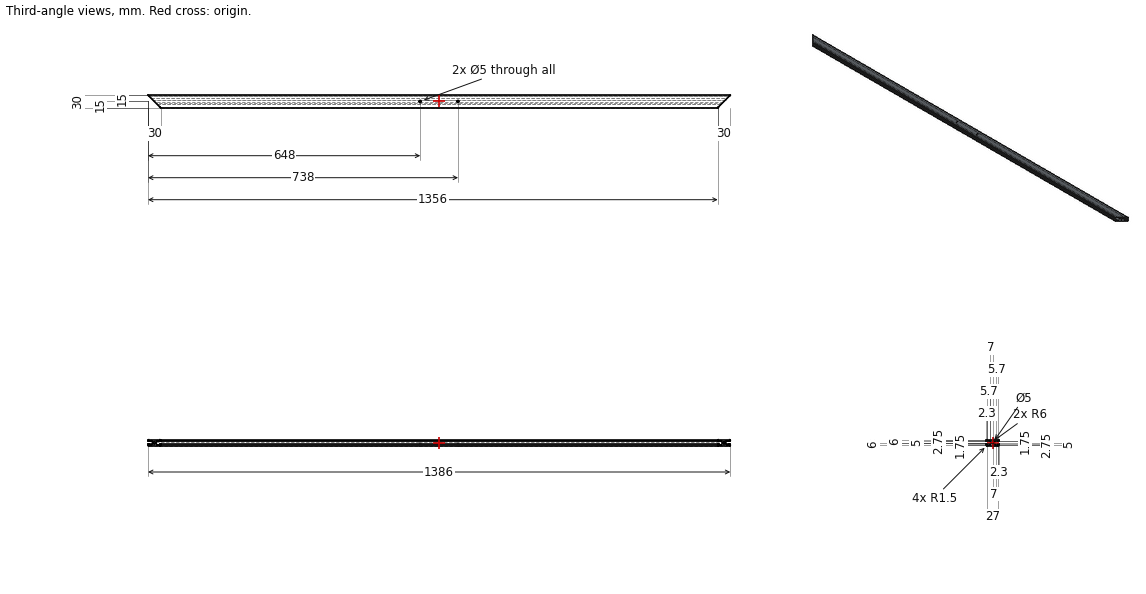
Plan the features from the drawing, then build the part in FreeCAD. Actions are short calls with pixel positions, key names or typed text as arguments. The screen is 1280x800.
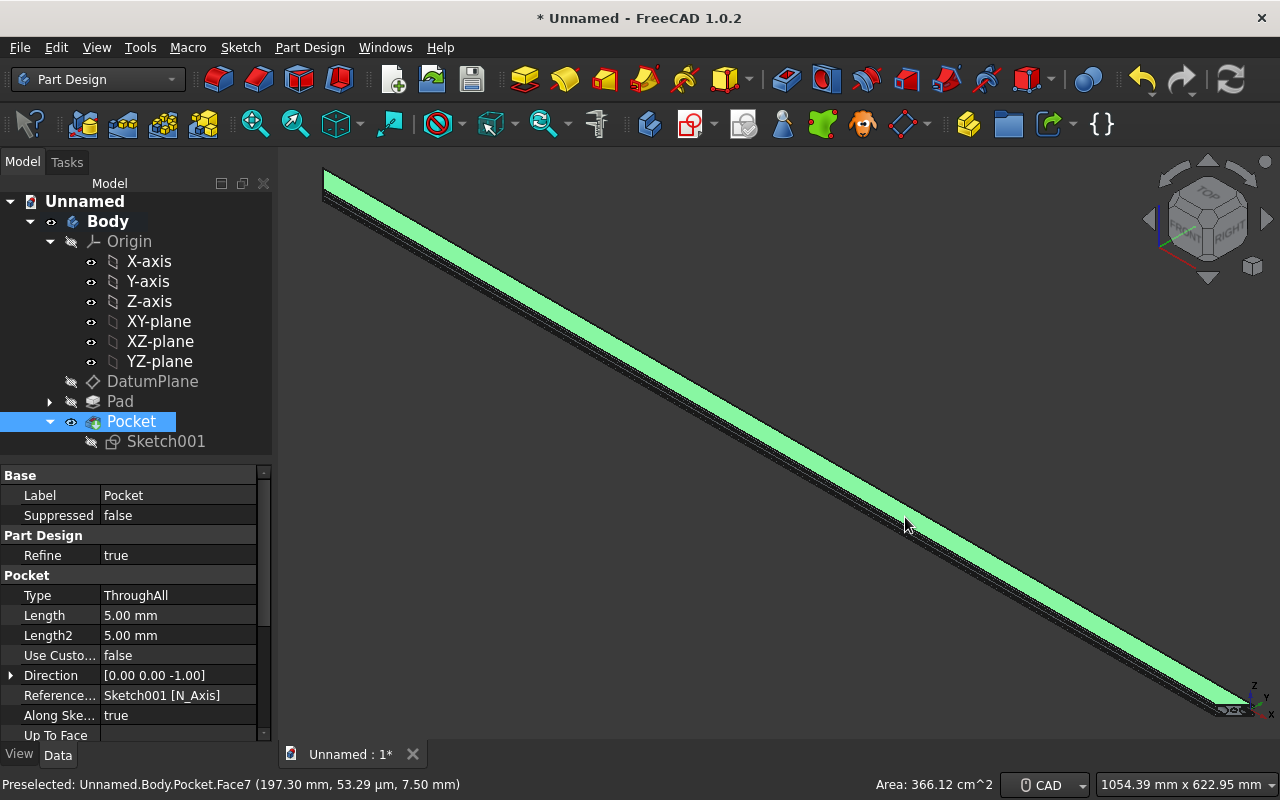
click(690, 124)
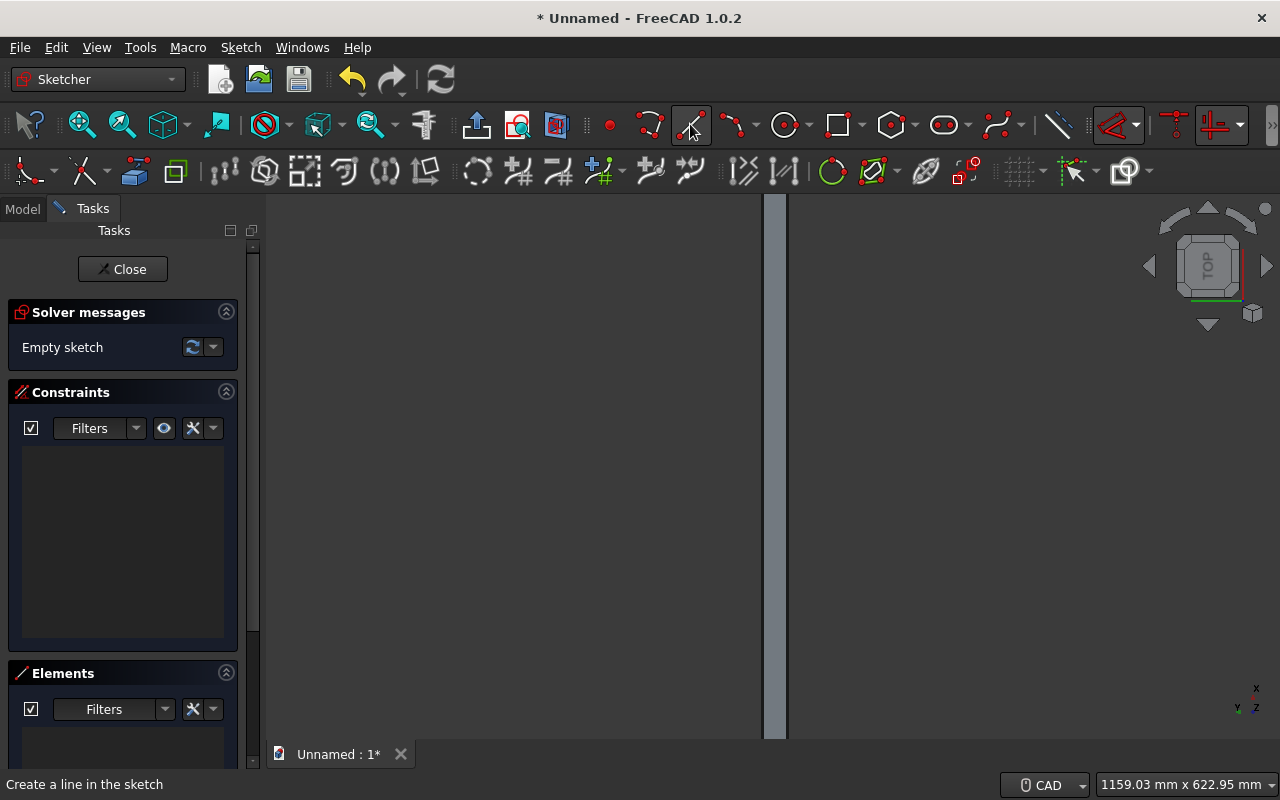
scroll(798, 465, up, 7)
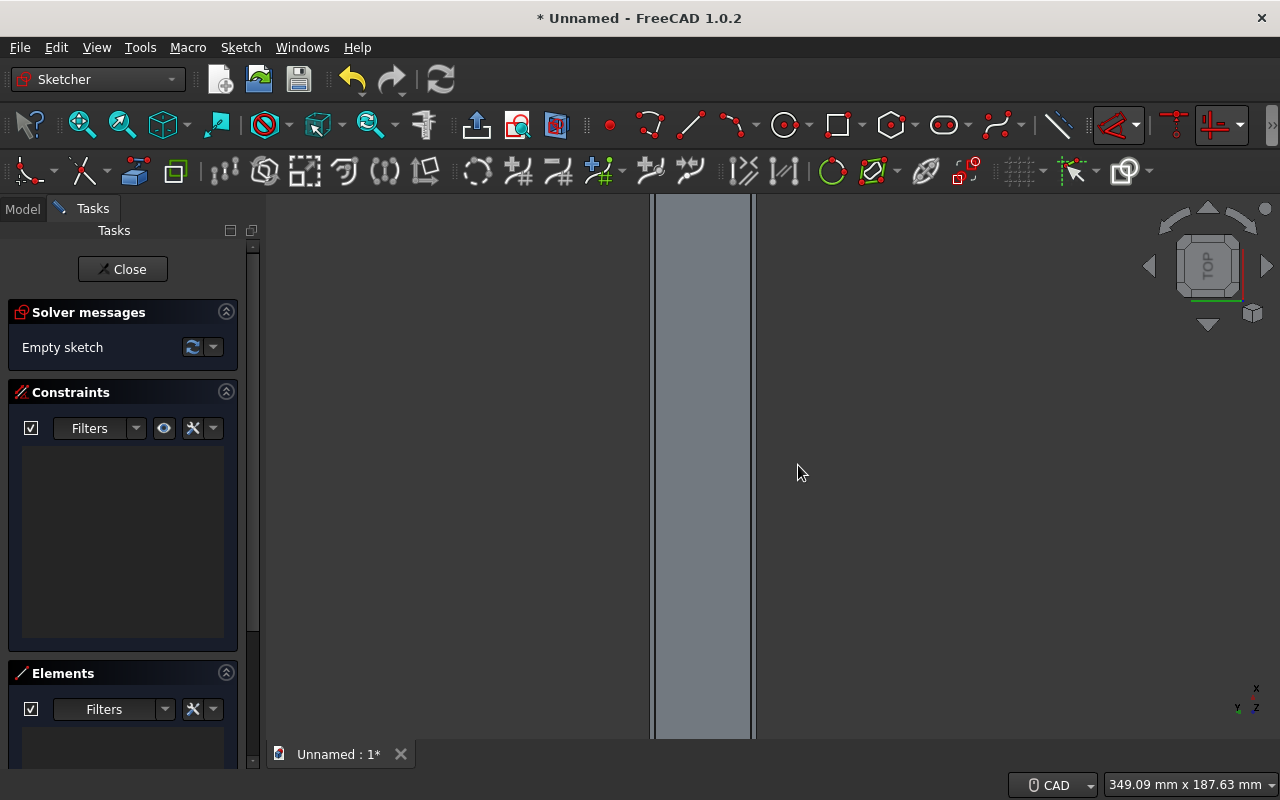
click(786, 126)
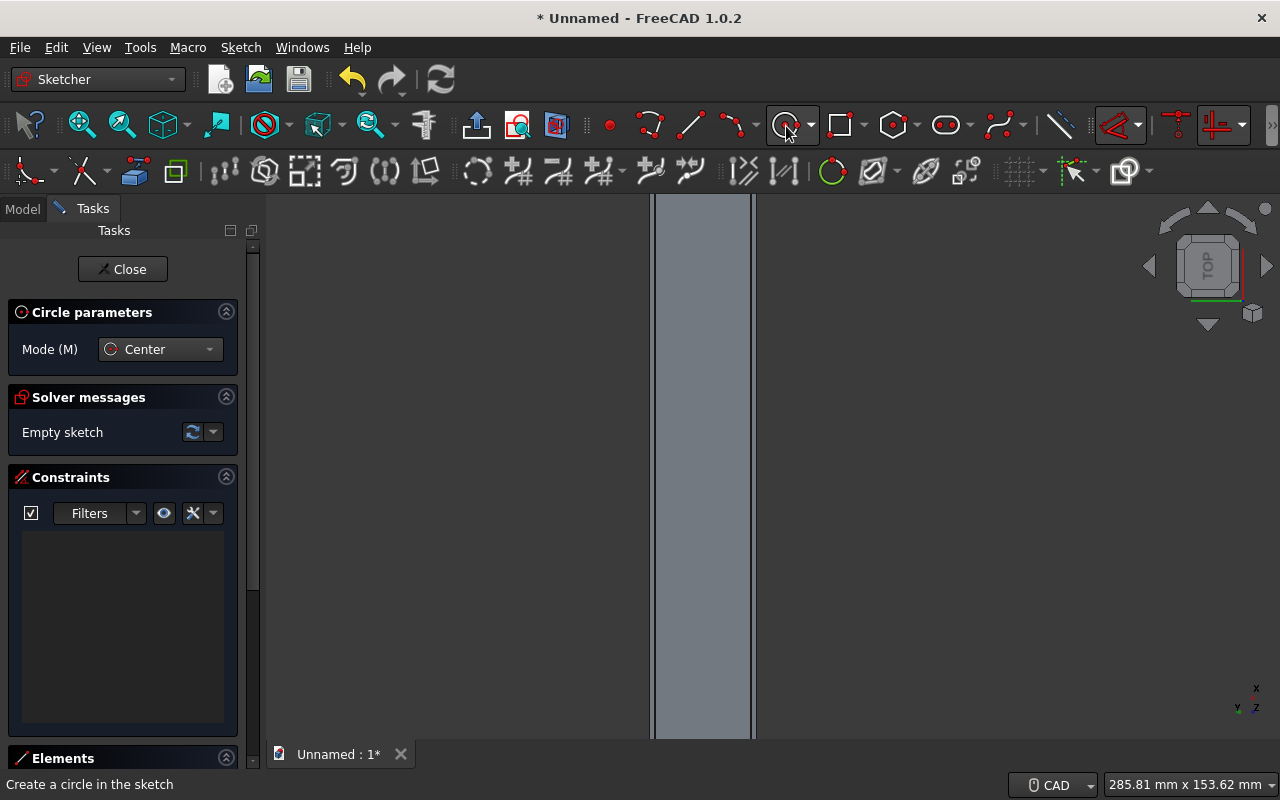
scroll(703, 624, up, 5)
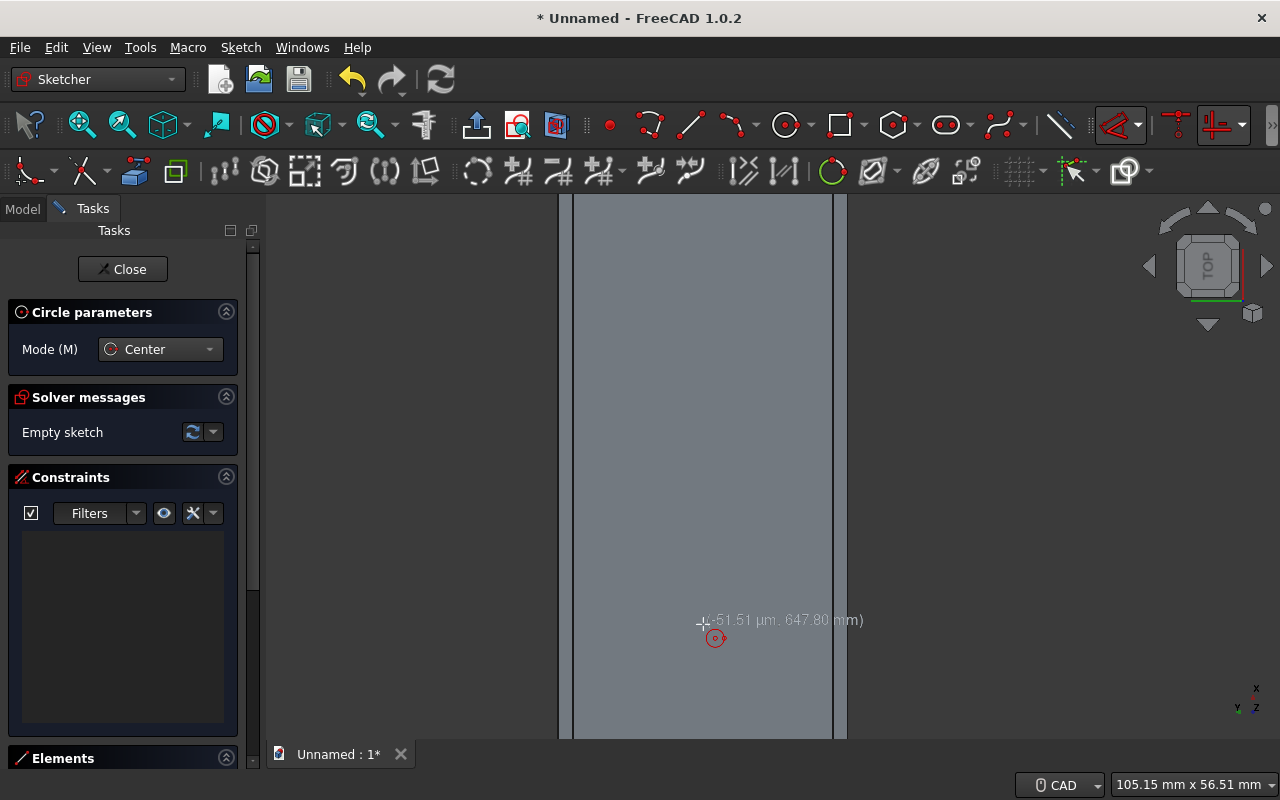
click(703, 623)
click(720, 606)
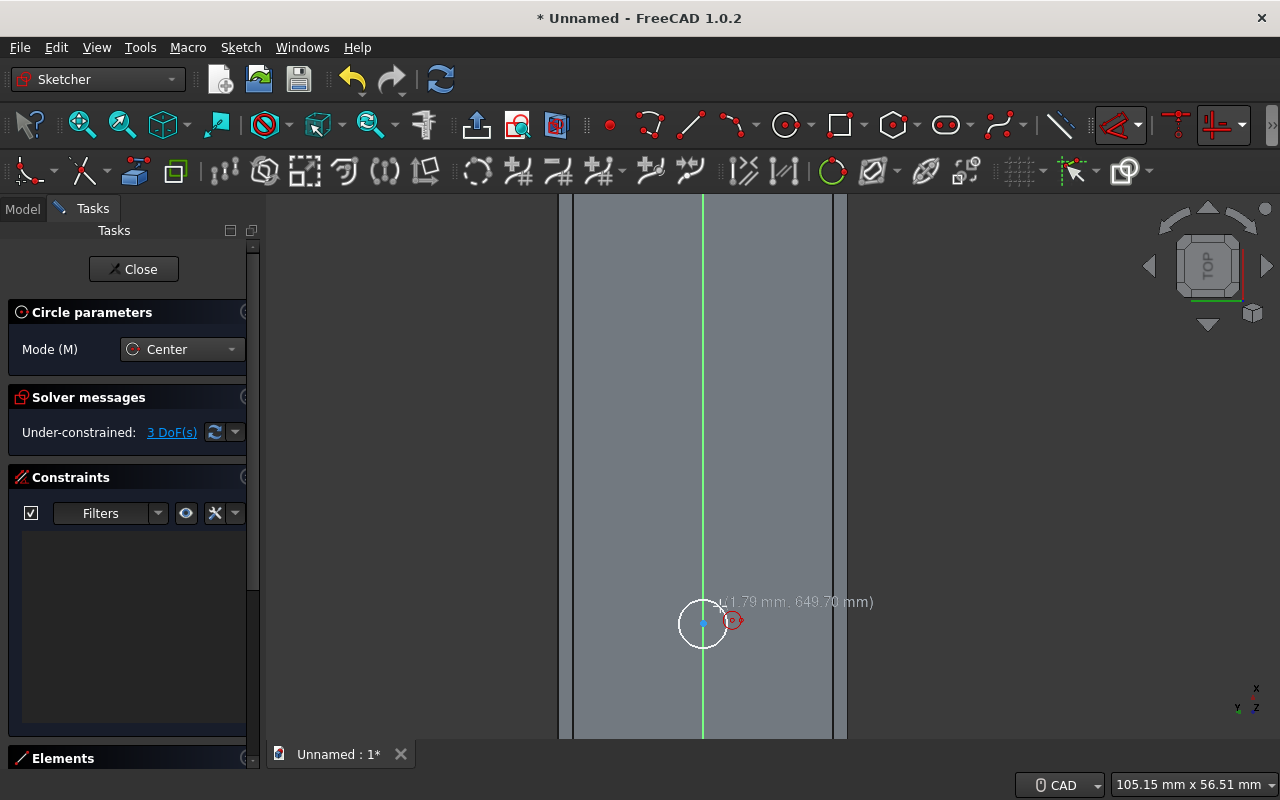
scroll(706, 628, down, 5)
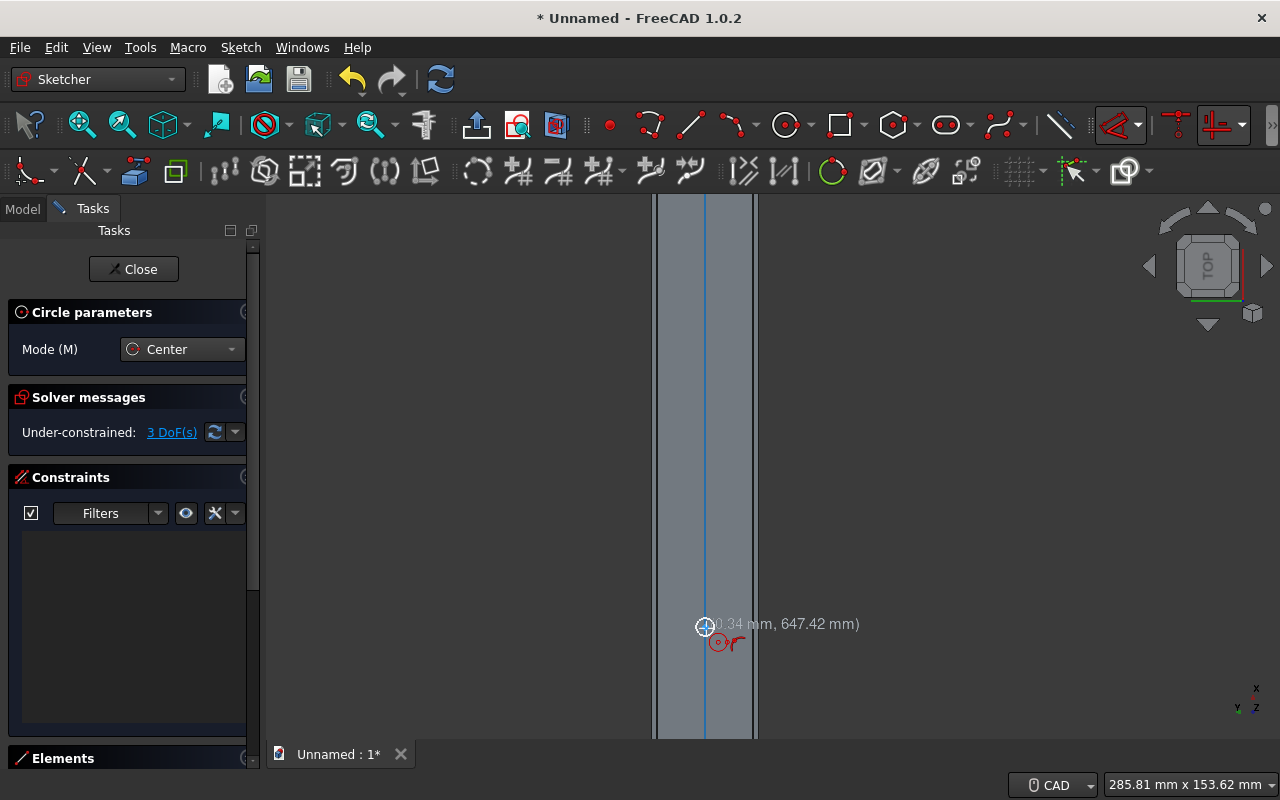
scroll(705, 308, up, 5)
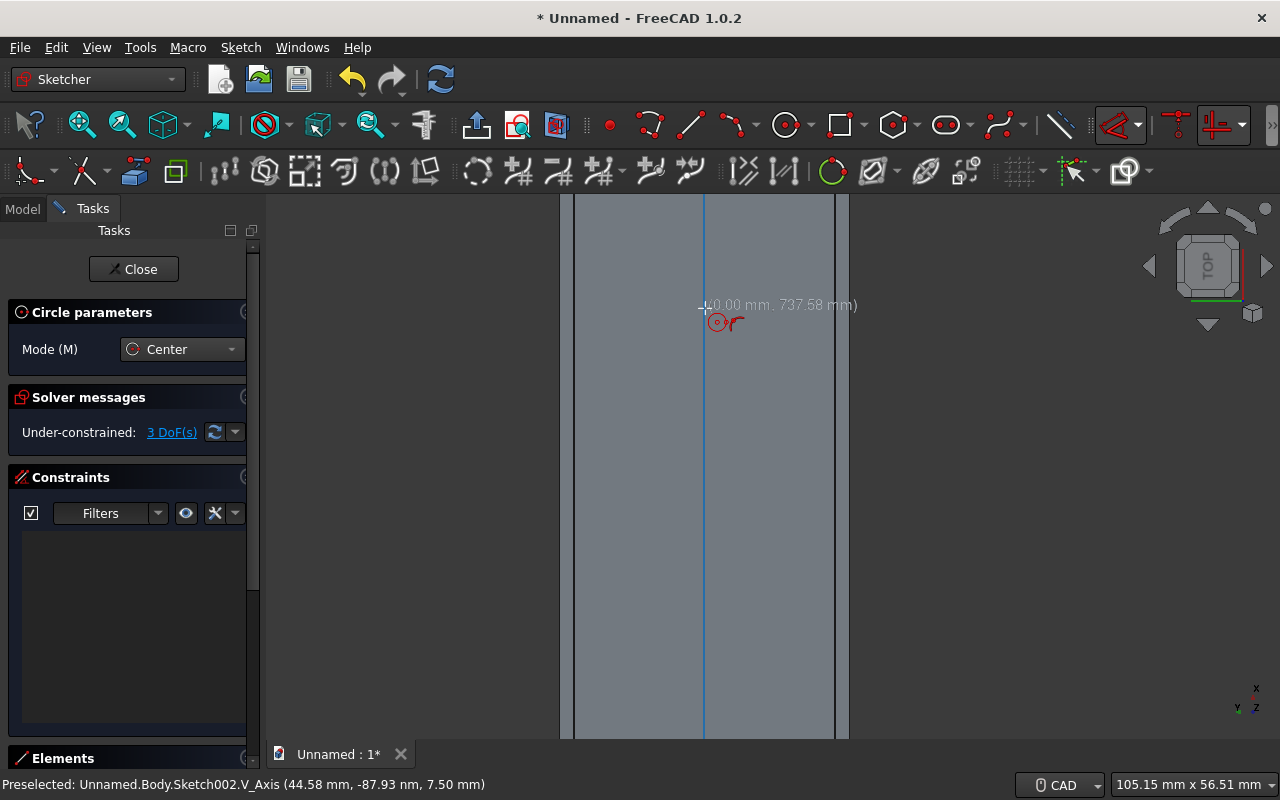
click(704, 306)
click(722, 289)
key(Escape)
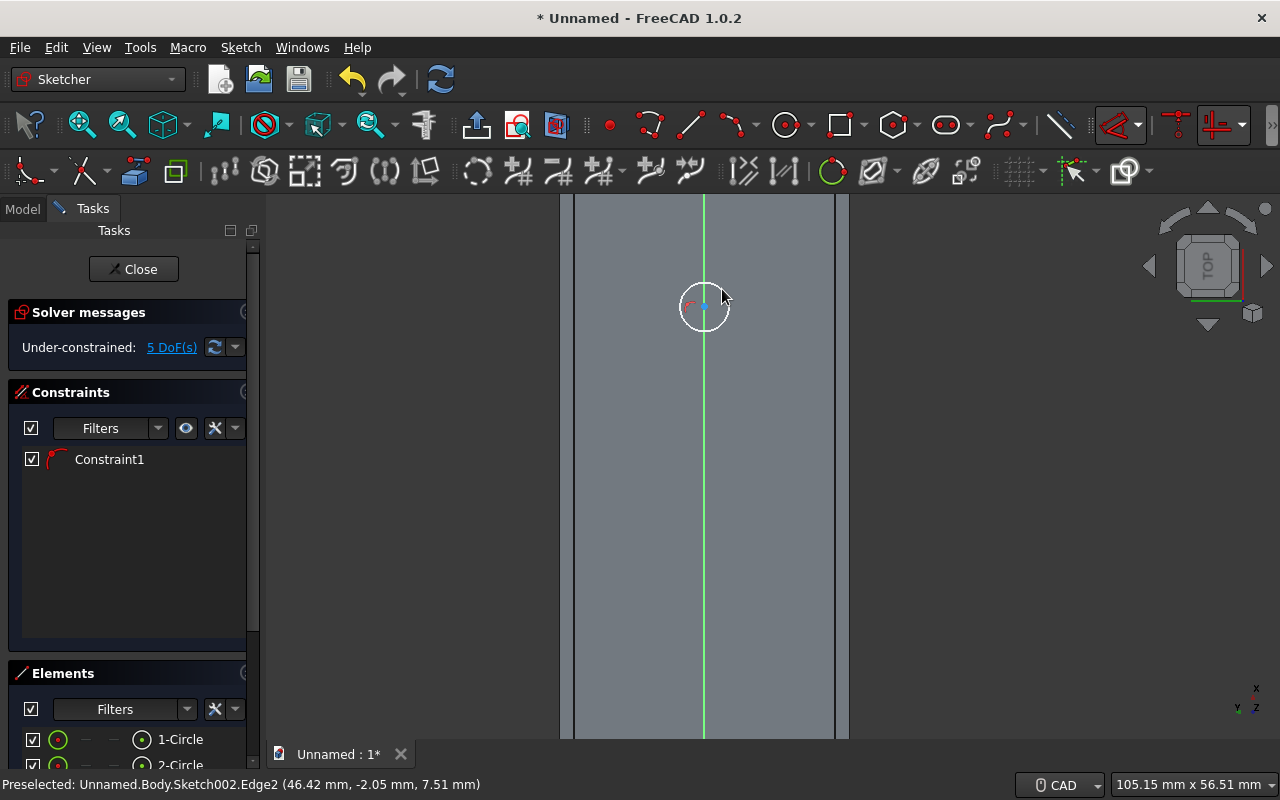
scroll(705, 307, down, 5)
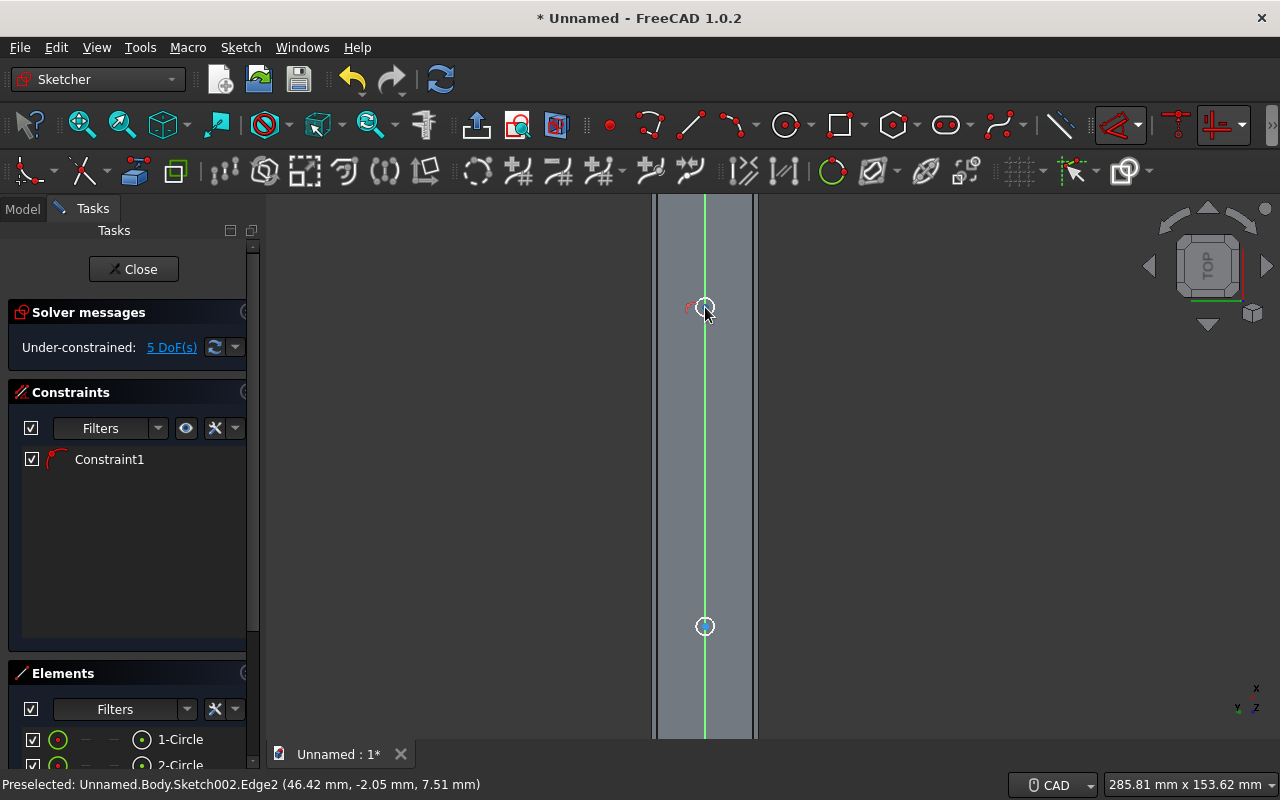
scroll(711, 620, up, 4)